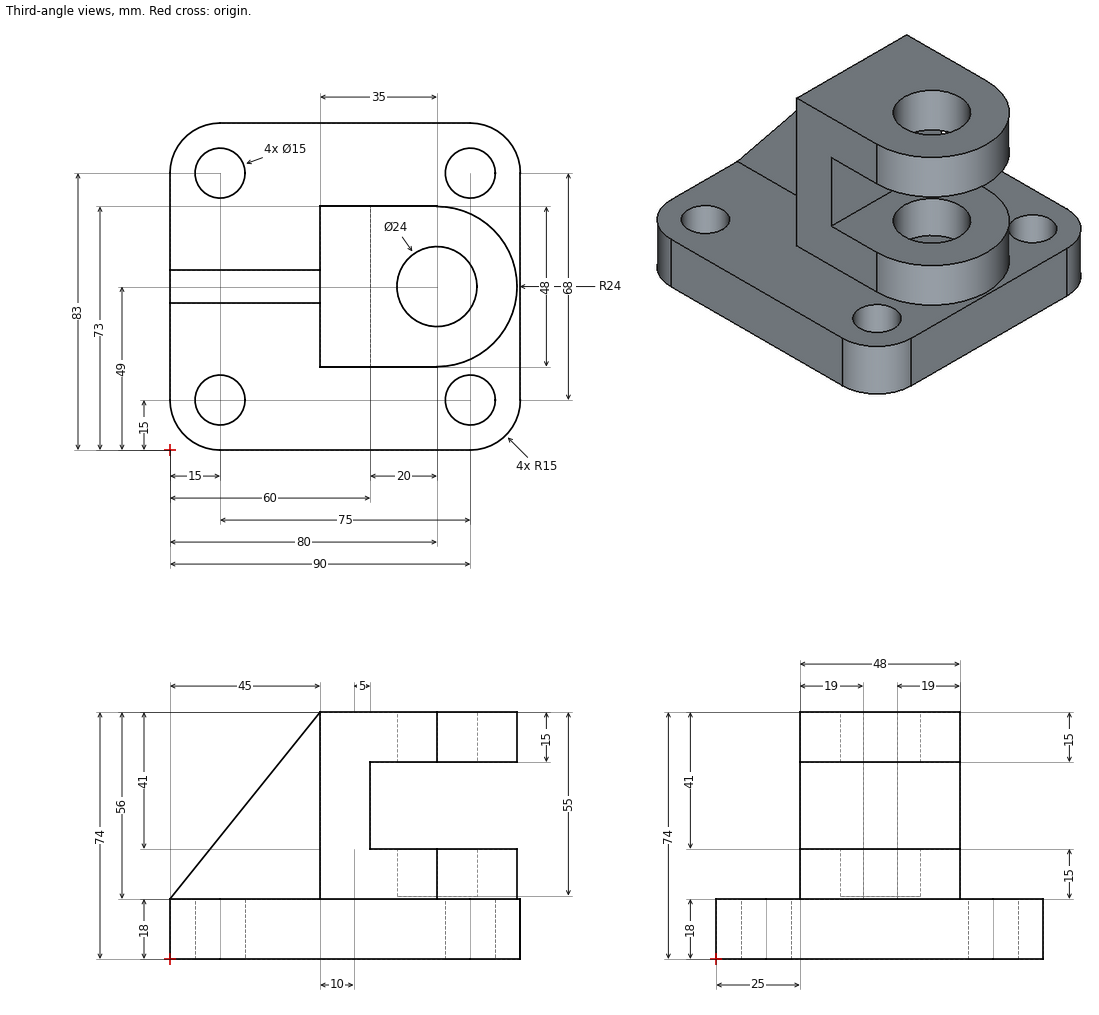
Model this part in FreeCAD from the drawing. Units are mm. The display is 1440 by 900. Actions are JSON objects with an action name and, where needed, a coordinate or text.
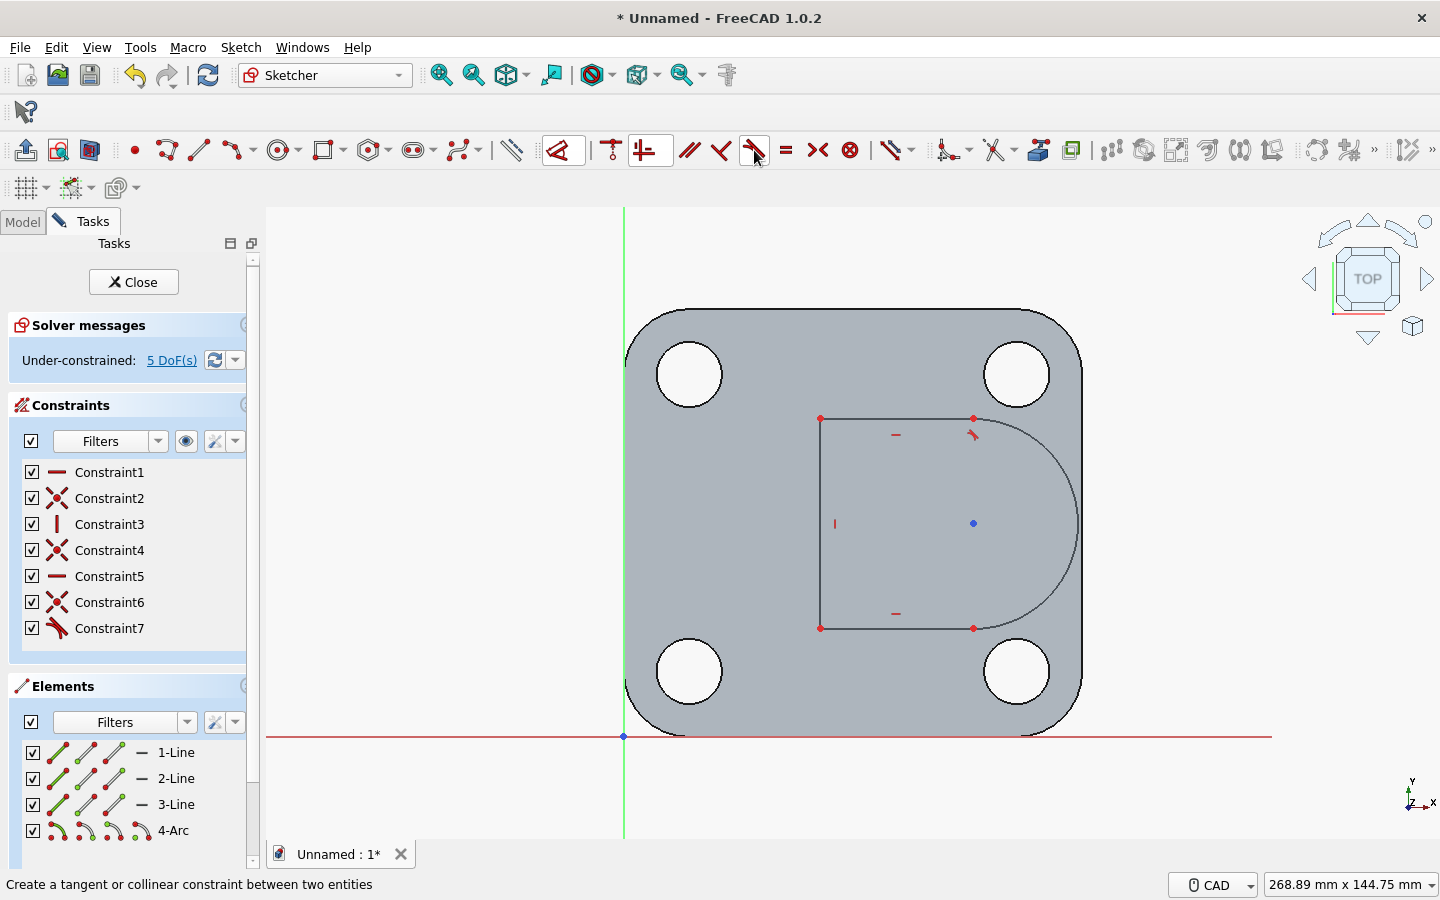
{"action": "left_click", "coordinate": [866, 629]}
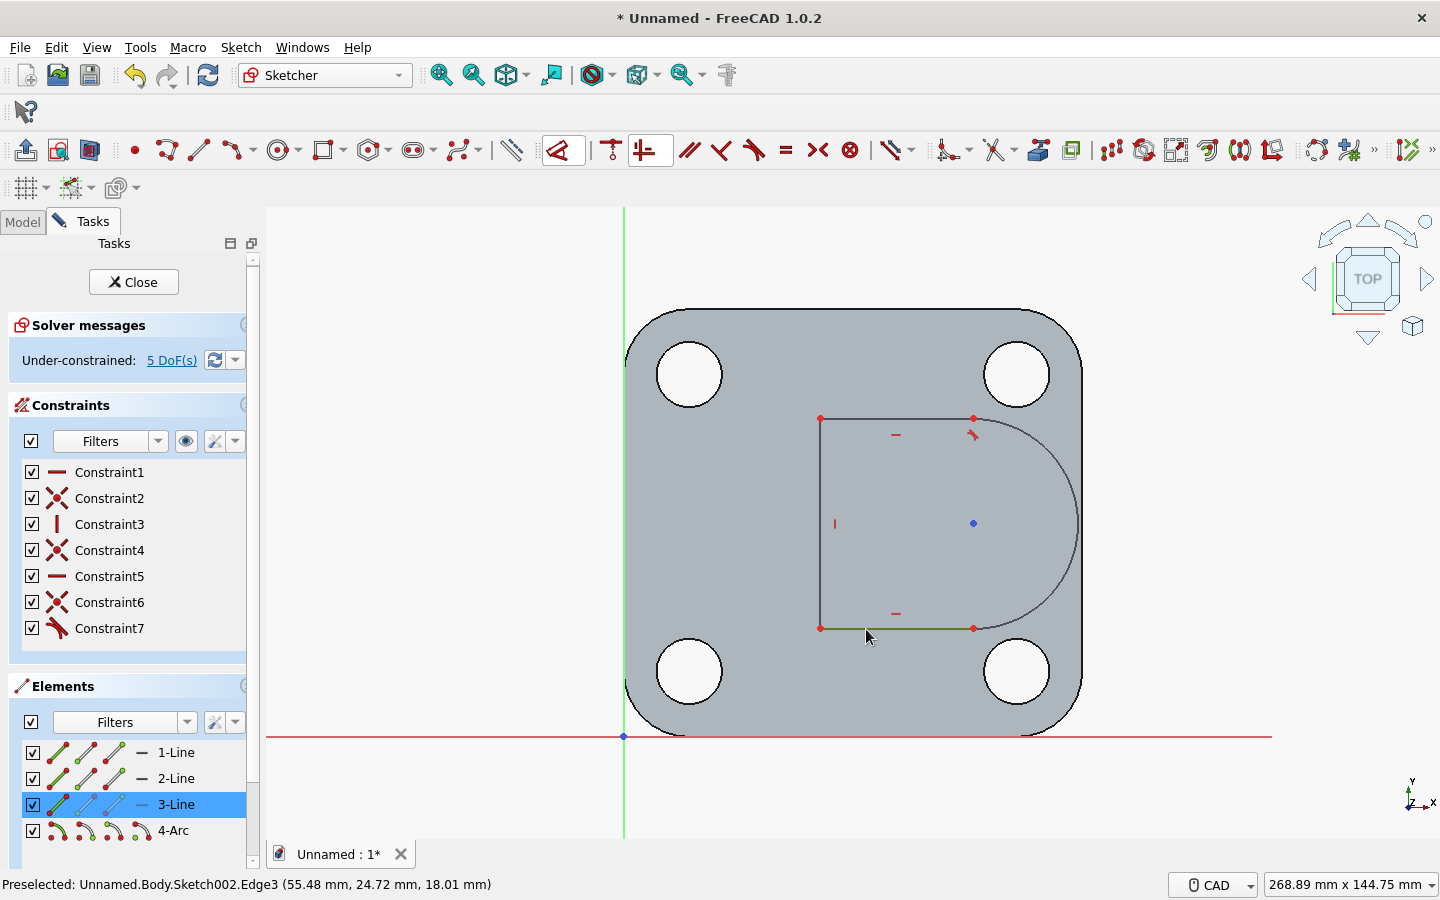
{"action": "left_click", "coordinate": [1058, 586]}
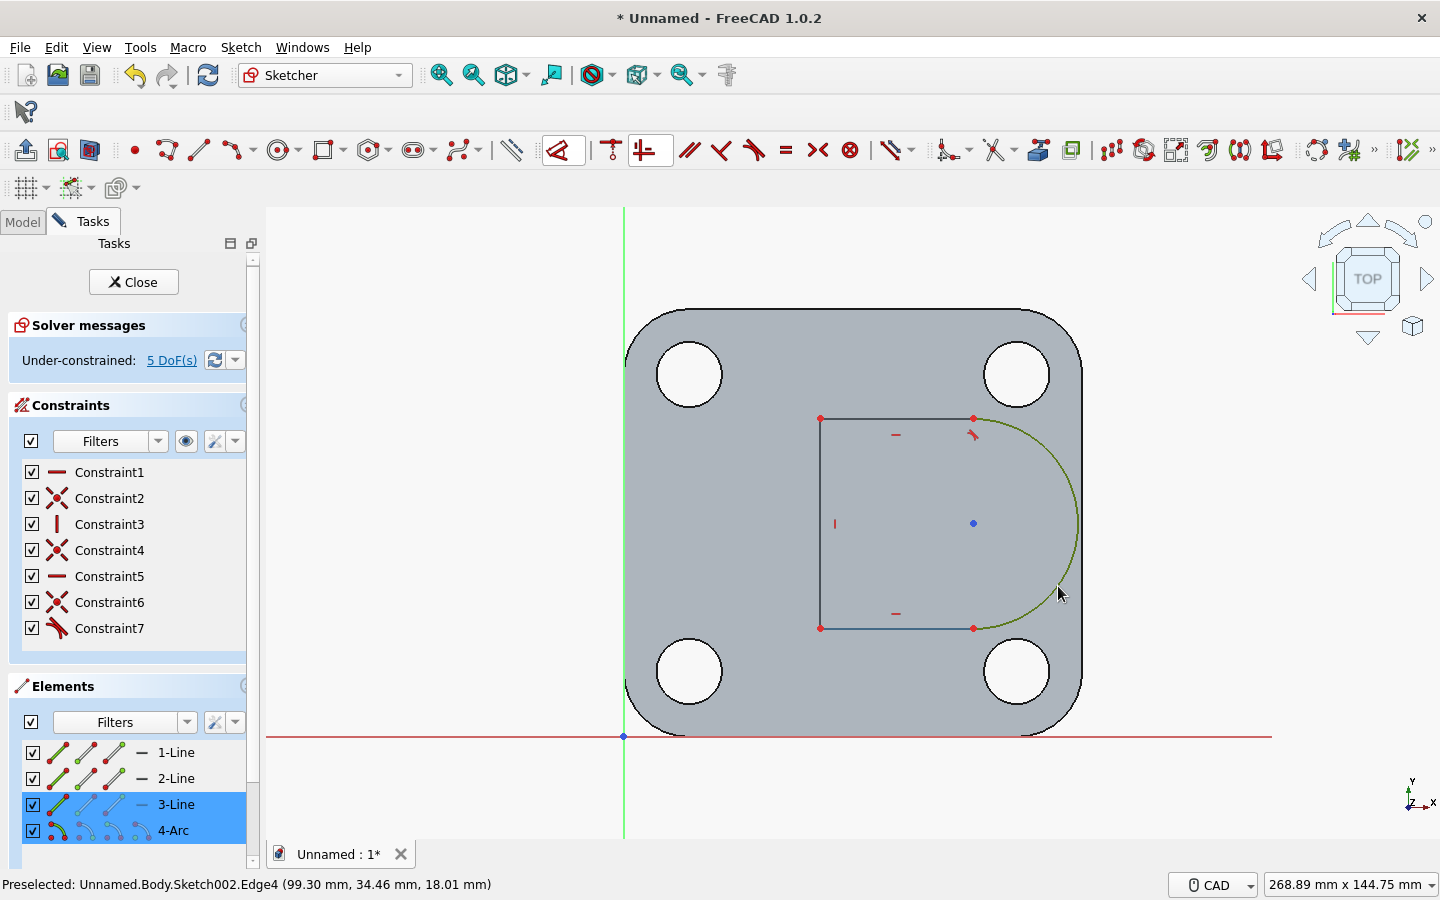
{"action": "left_click", "coordinate": [754, 150]}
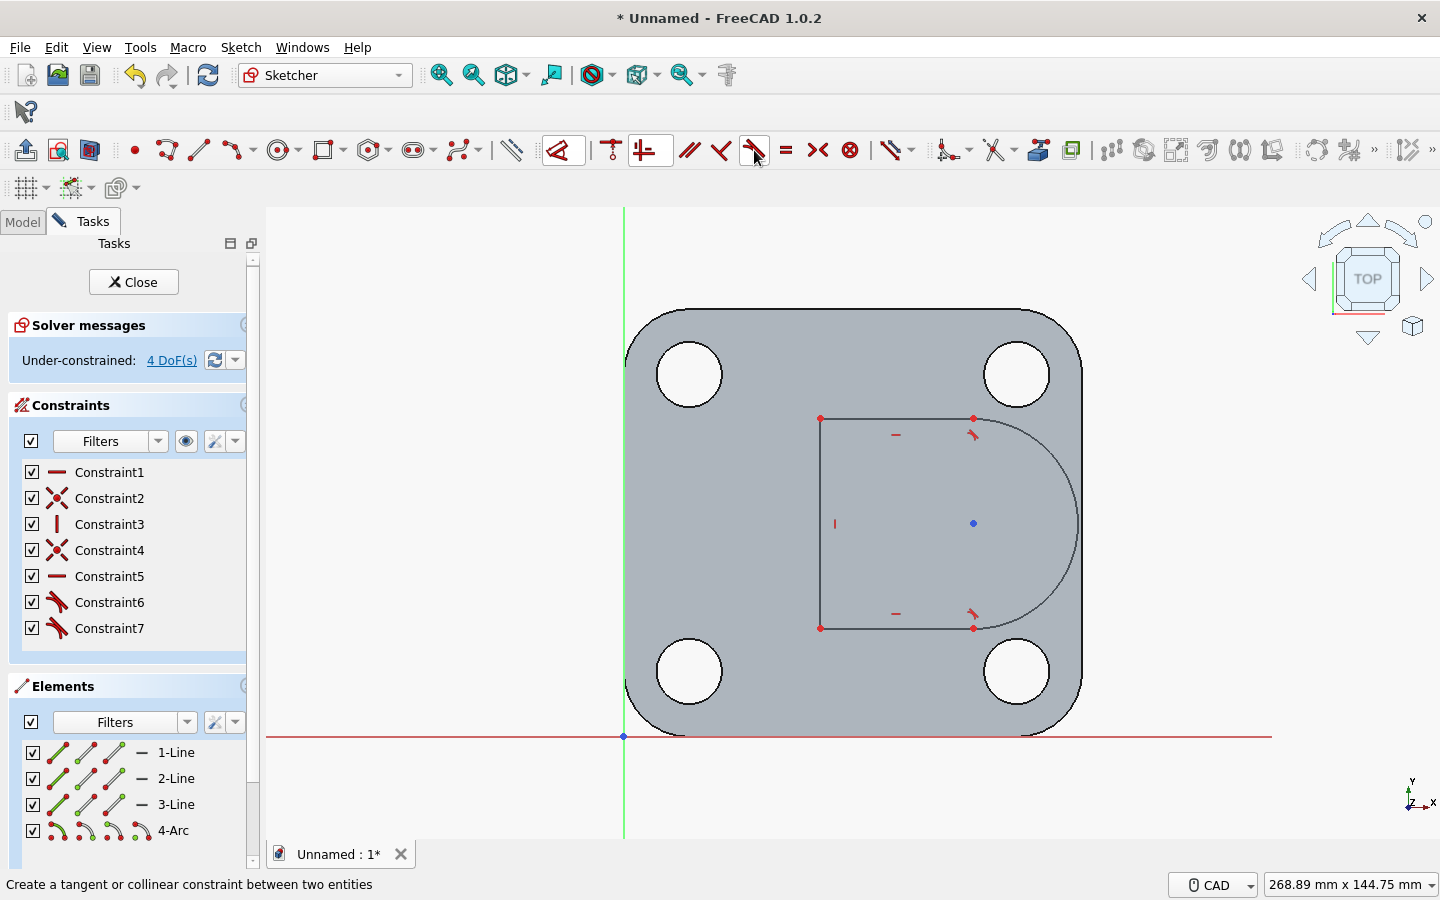
{"action": "left_click", "coordinate": [1058, 586]}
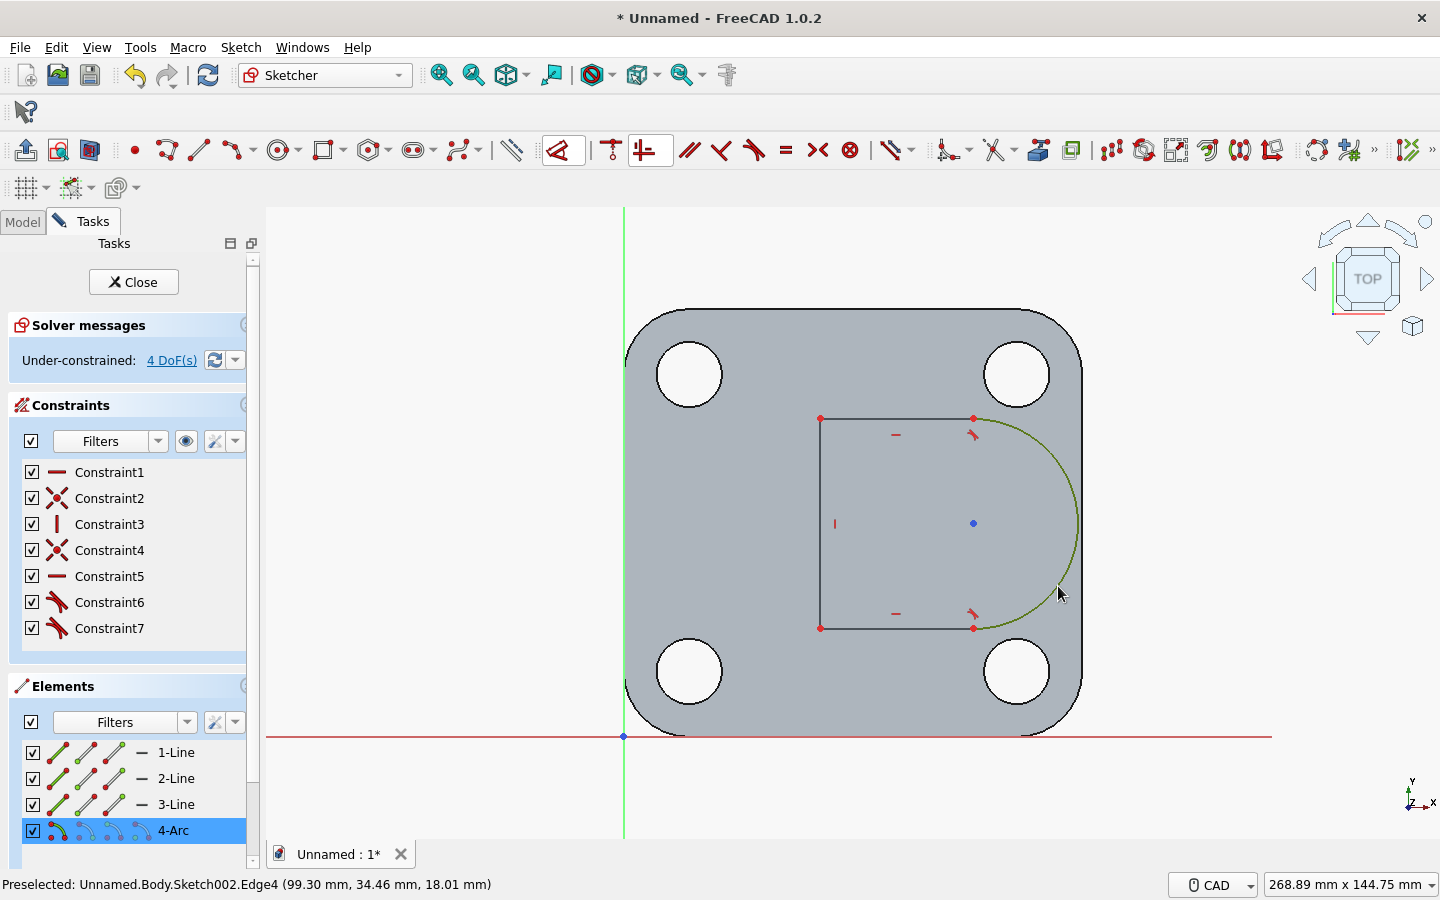
{"action": "key", "text": "k r"}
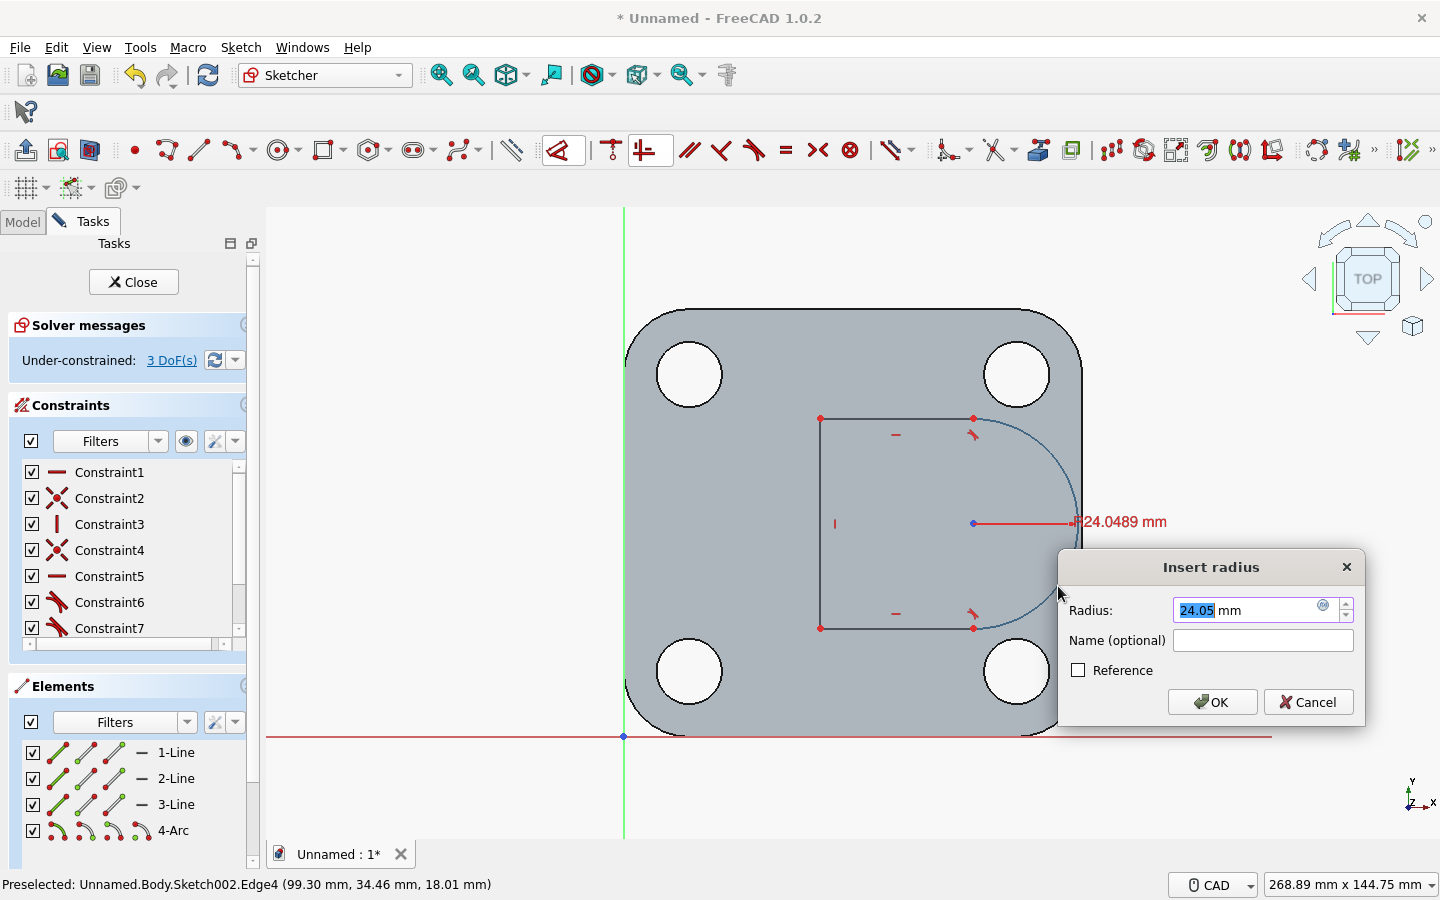
{"action": "type", "text": "24"}
{"action": "key", "text": "Return"}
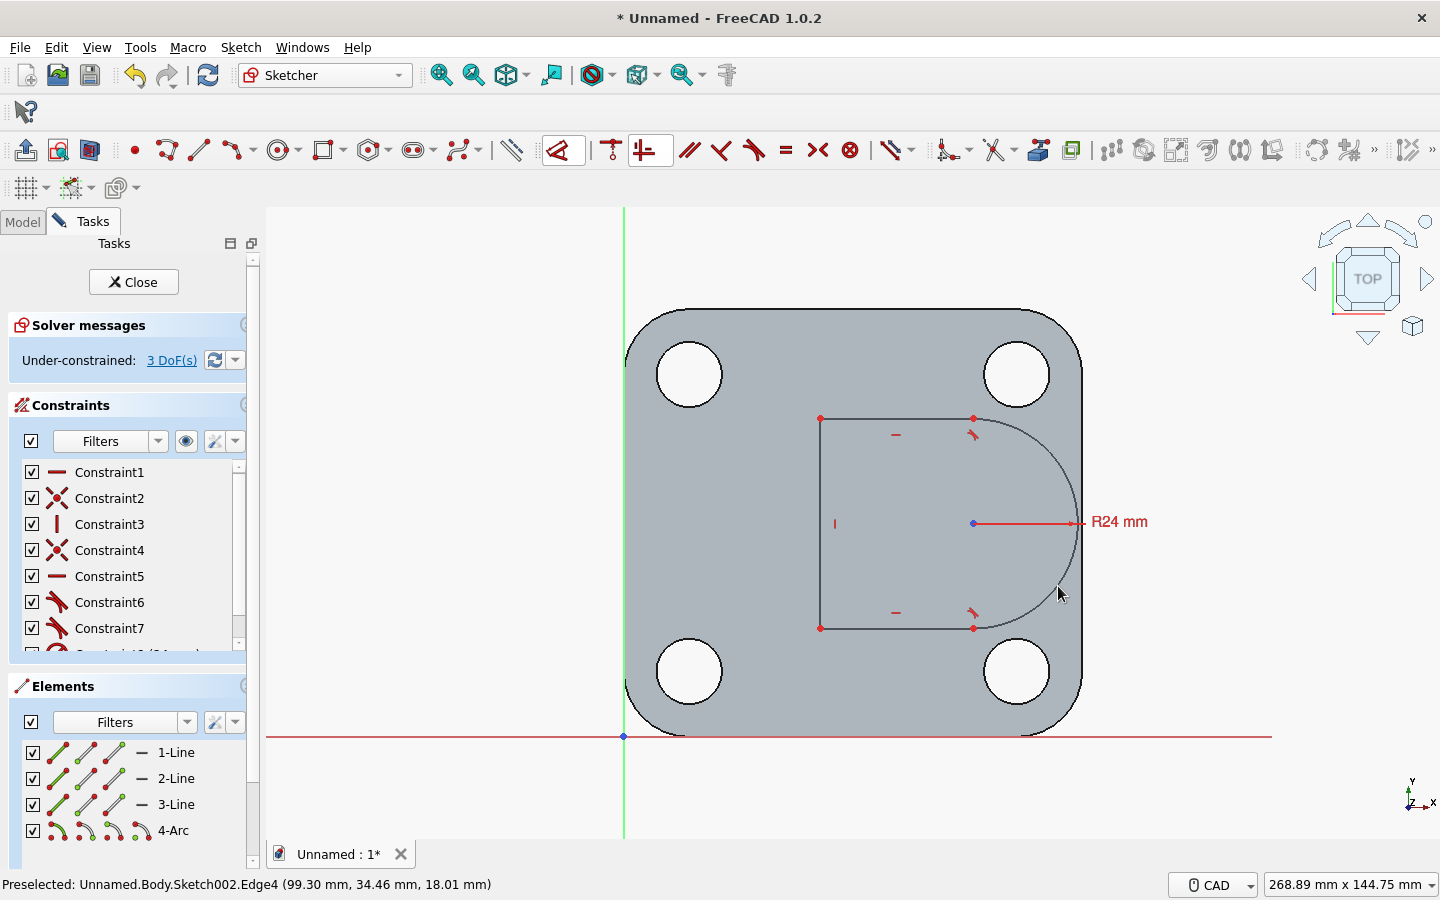
{"action": "left_click", "coordinate": [927, 419]}